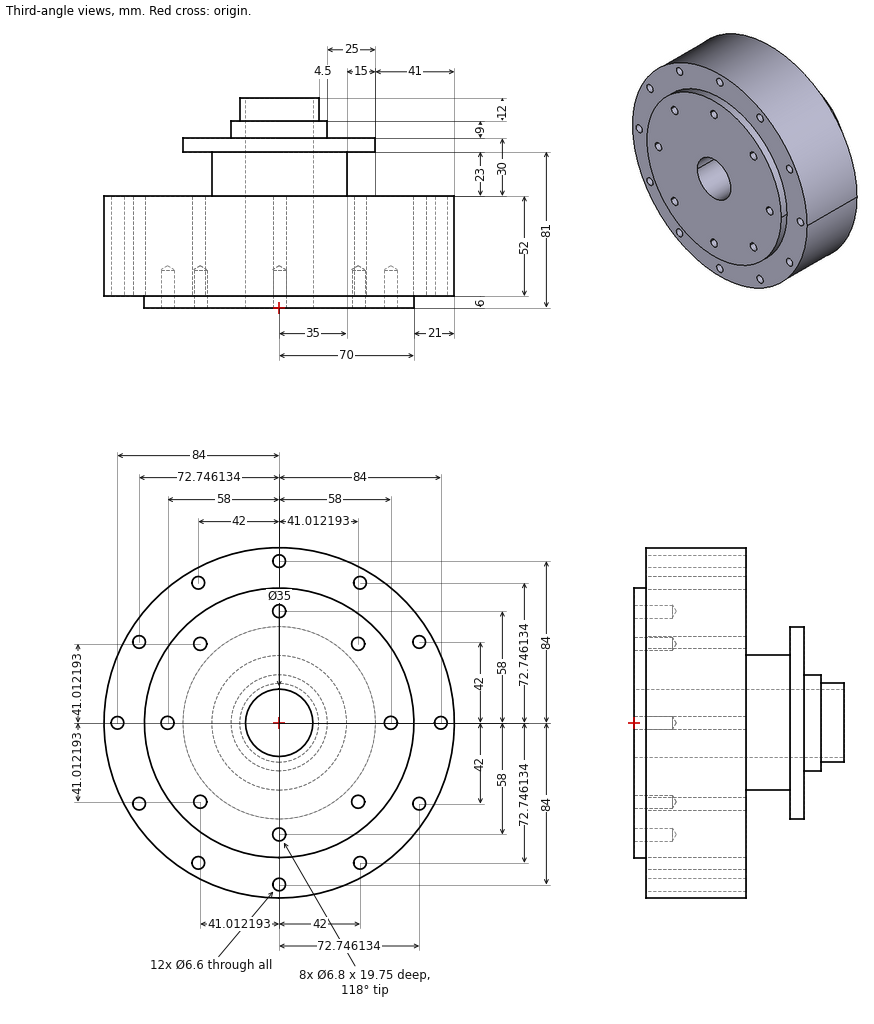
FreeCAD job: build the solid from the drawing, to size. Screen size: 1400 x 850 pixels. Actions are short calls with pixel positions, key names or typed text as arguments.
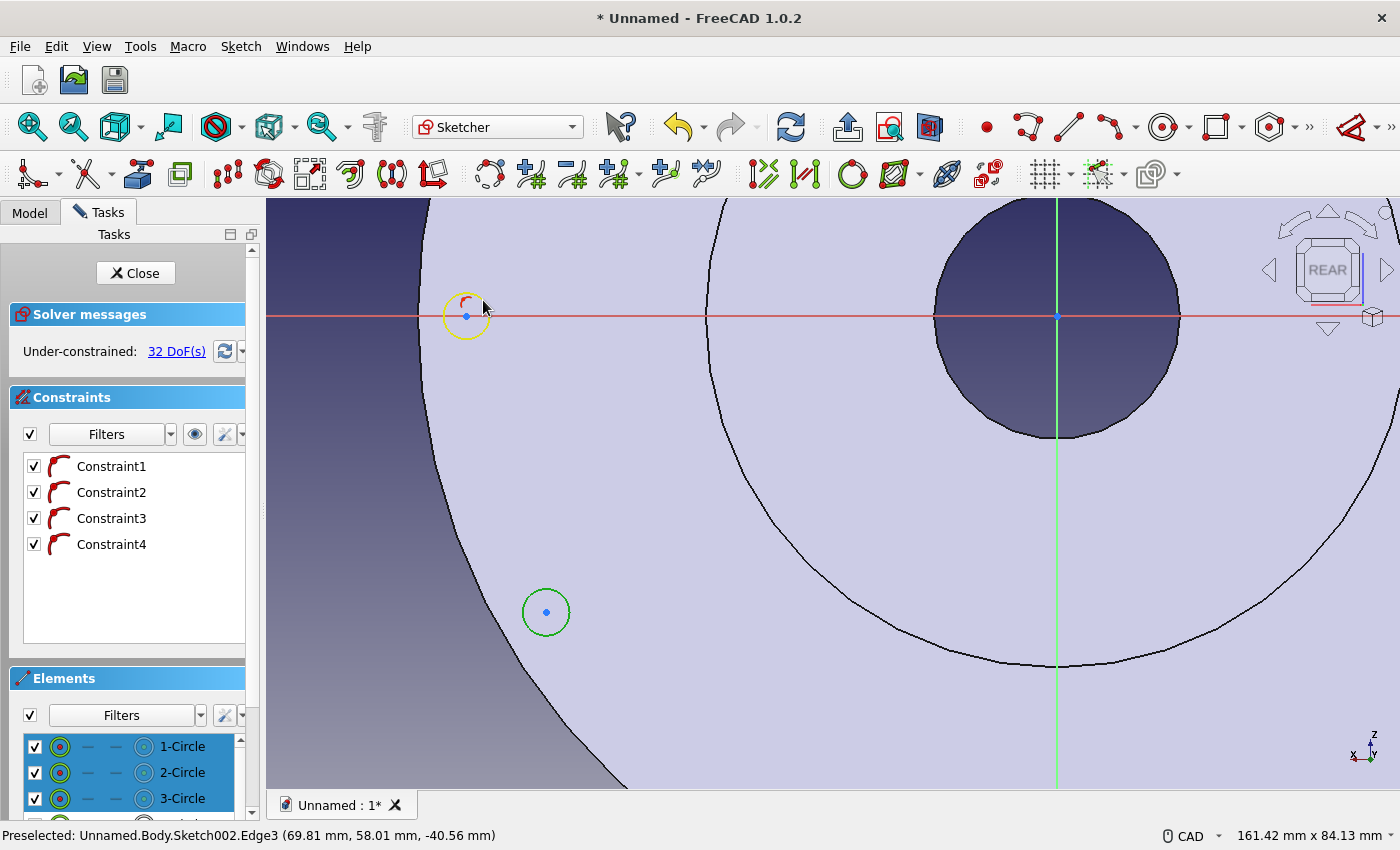
click(483, 300)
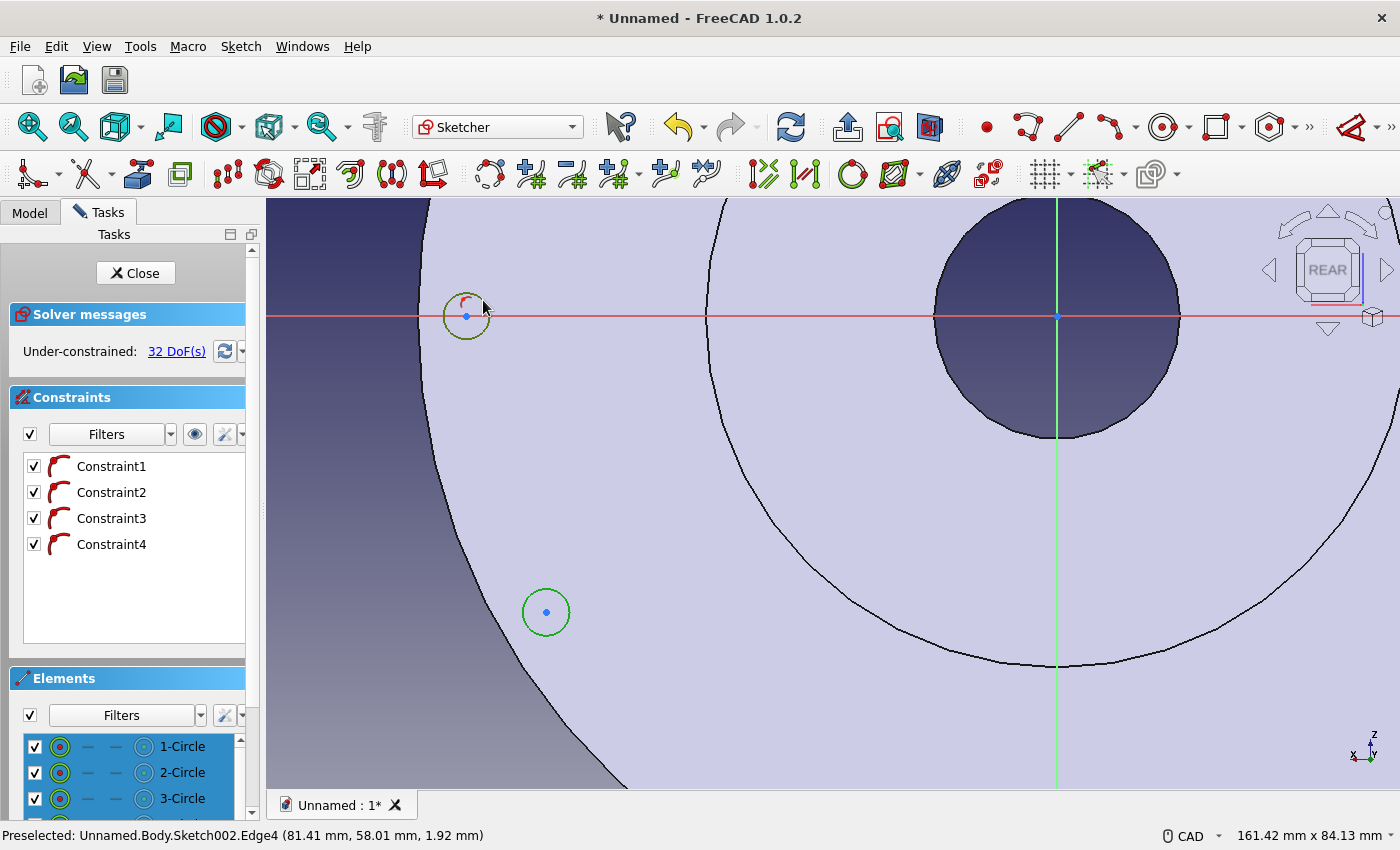
scroll(638, 570, down, 6)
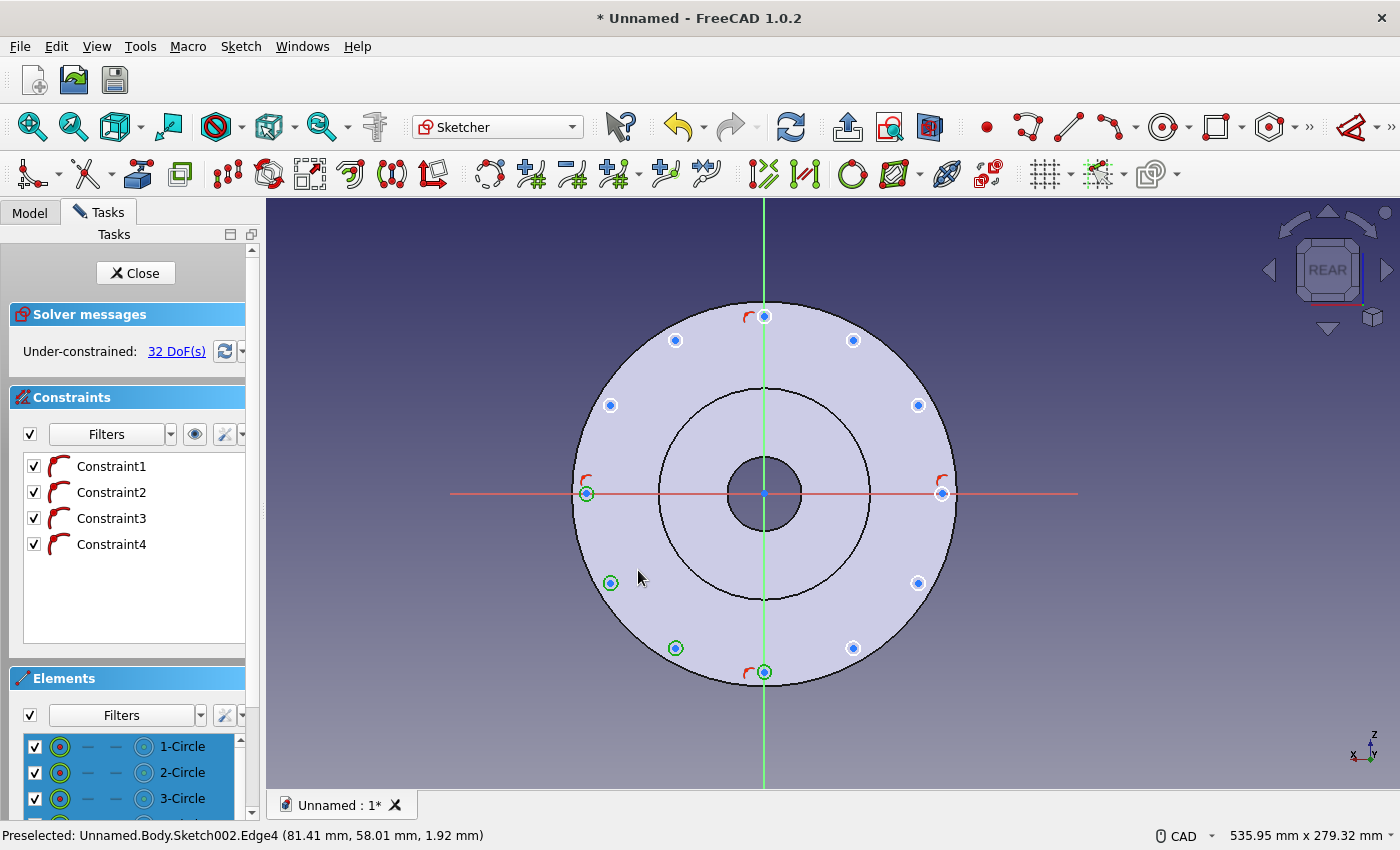
scroll(615, 401, up, 4)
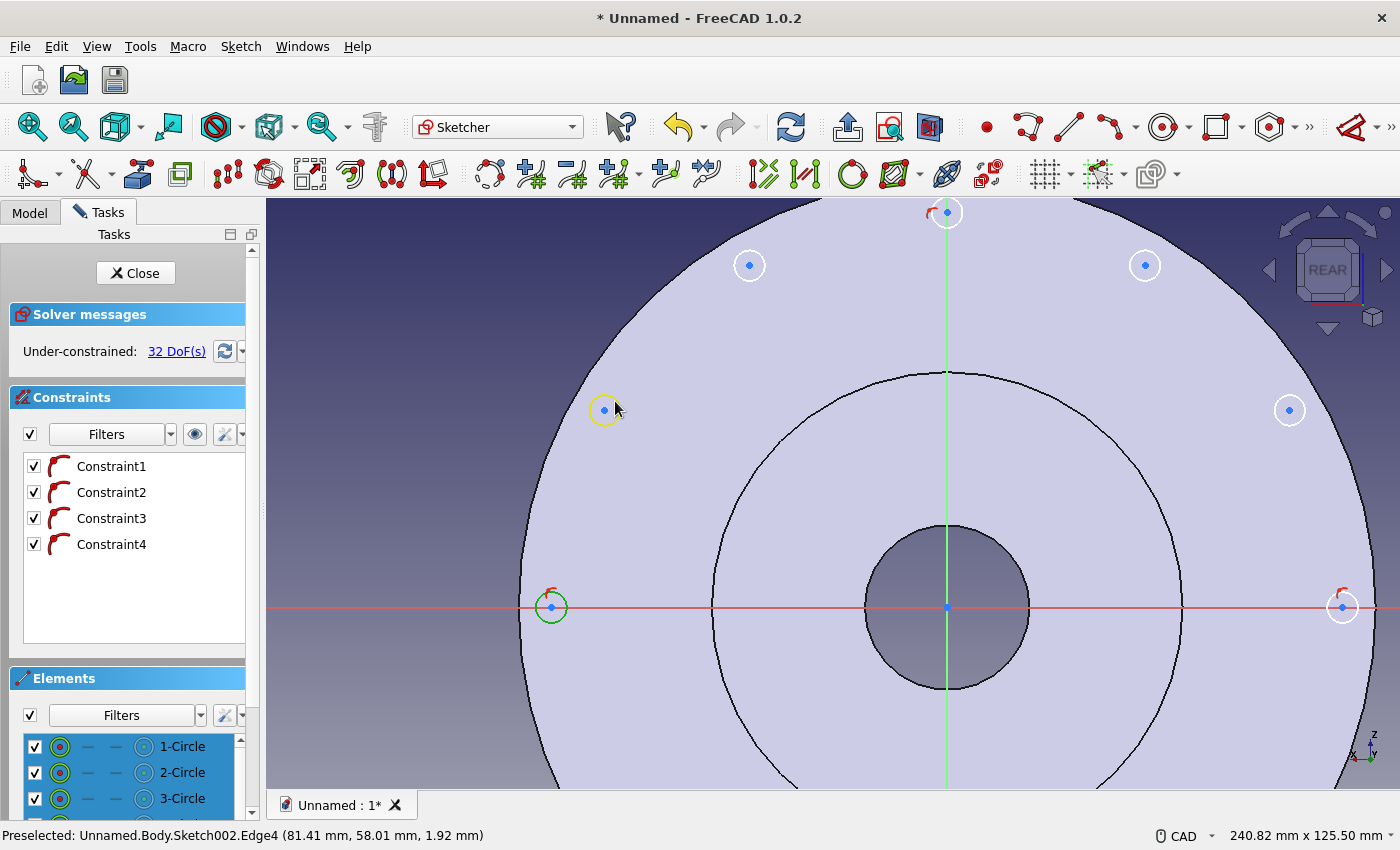
click(616, 400)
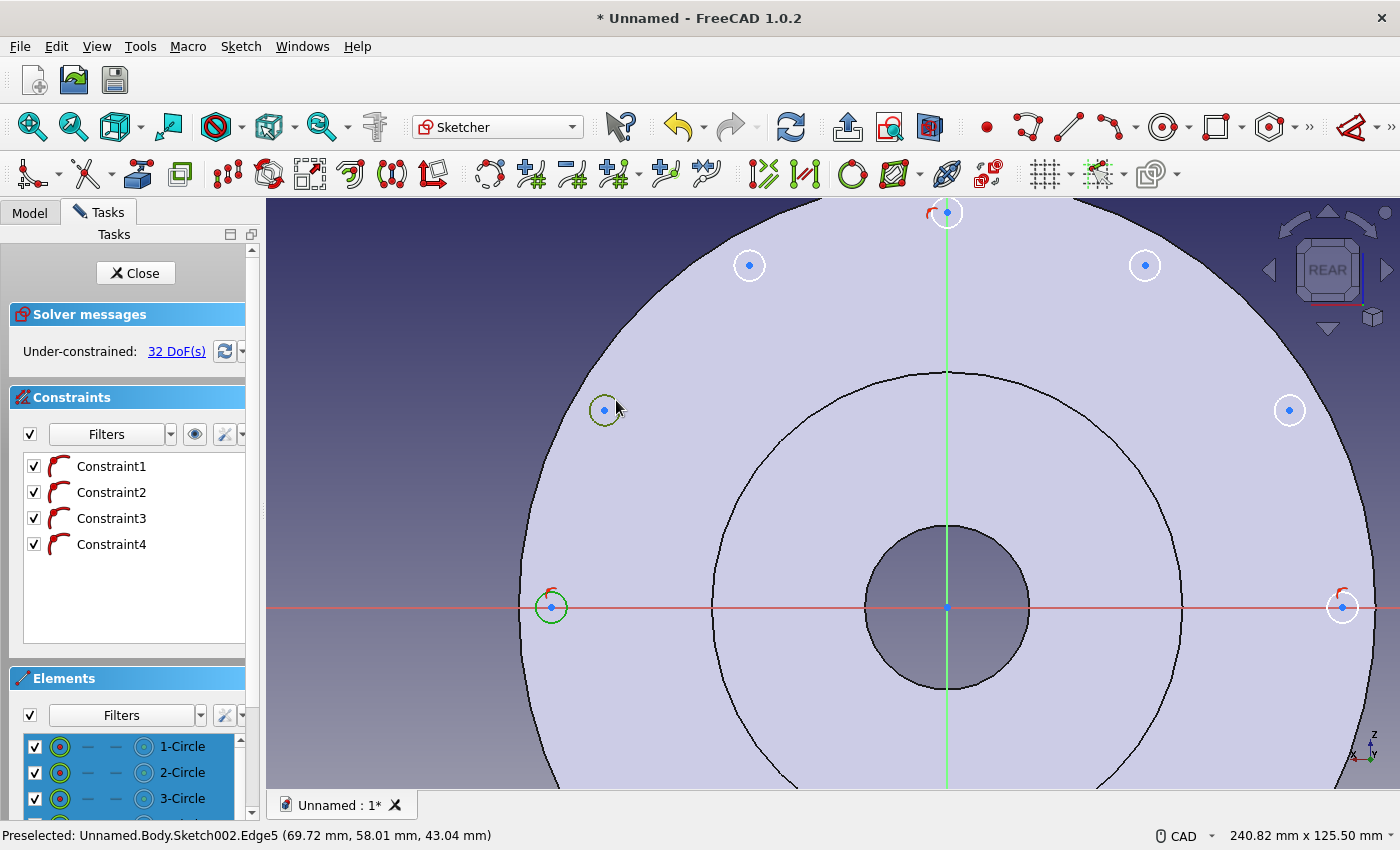
click(760, 255)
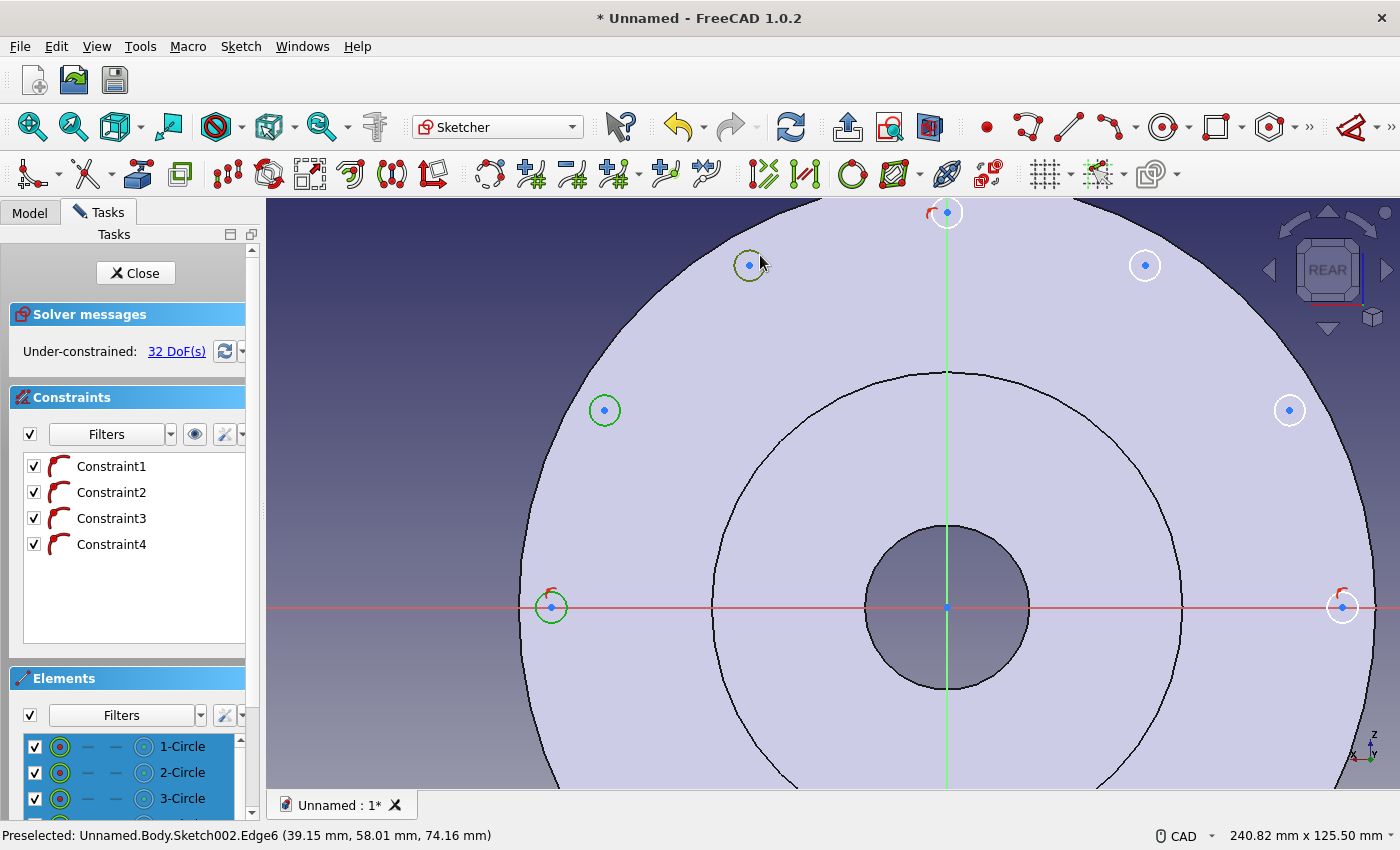
click(947, 228)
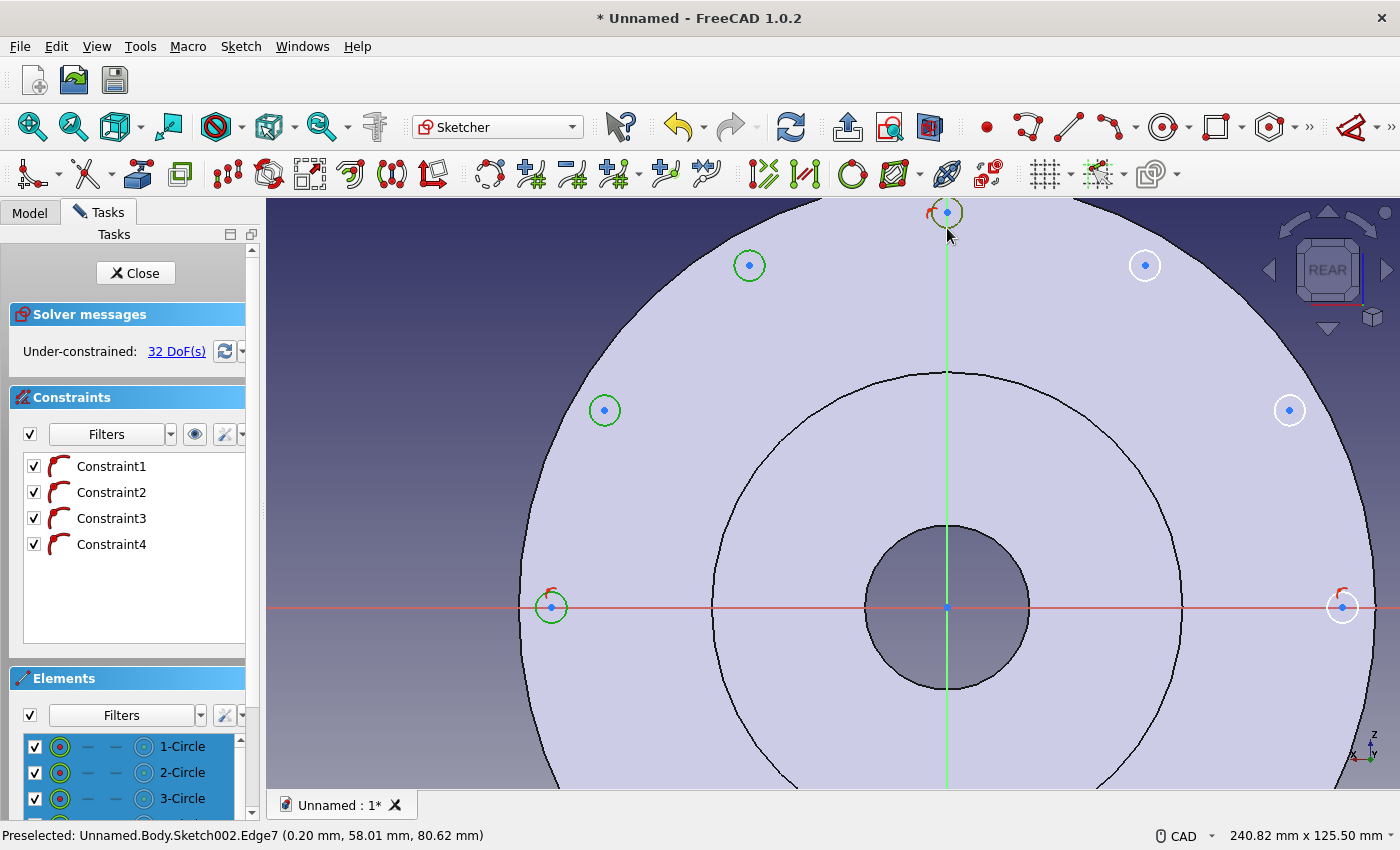
click(1156, 255)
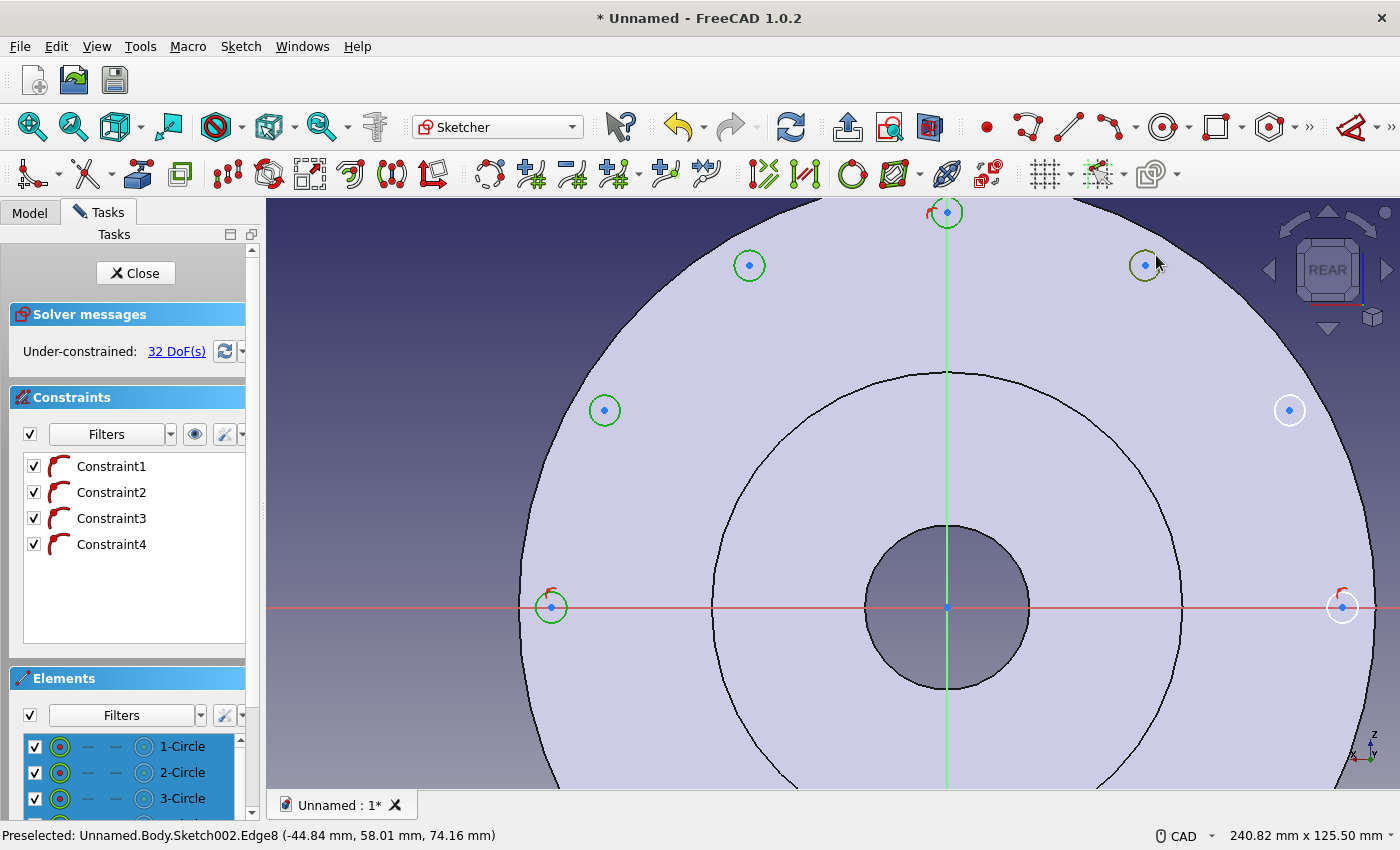
scroll(615, 400, down, 4)